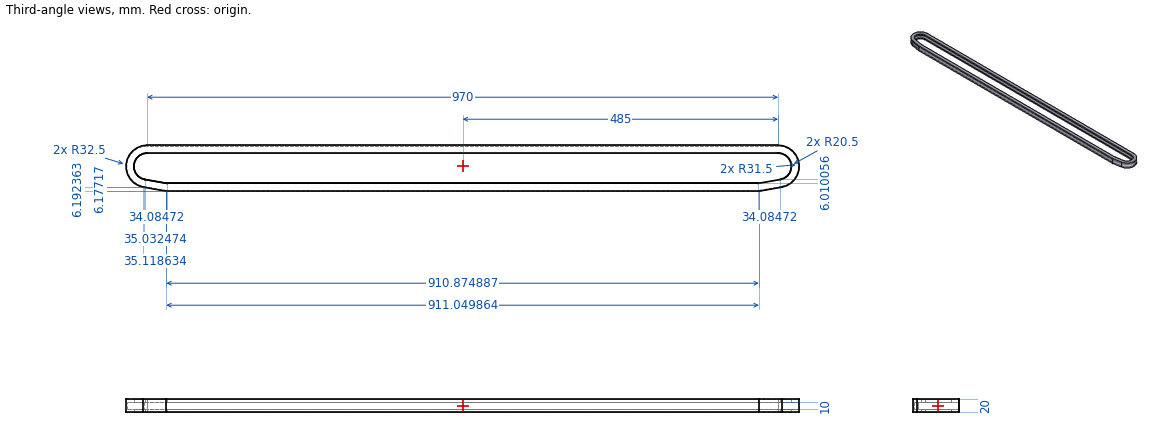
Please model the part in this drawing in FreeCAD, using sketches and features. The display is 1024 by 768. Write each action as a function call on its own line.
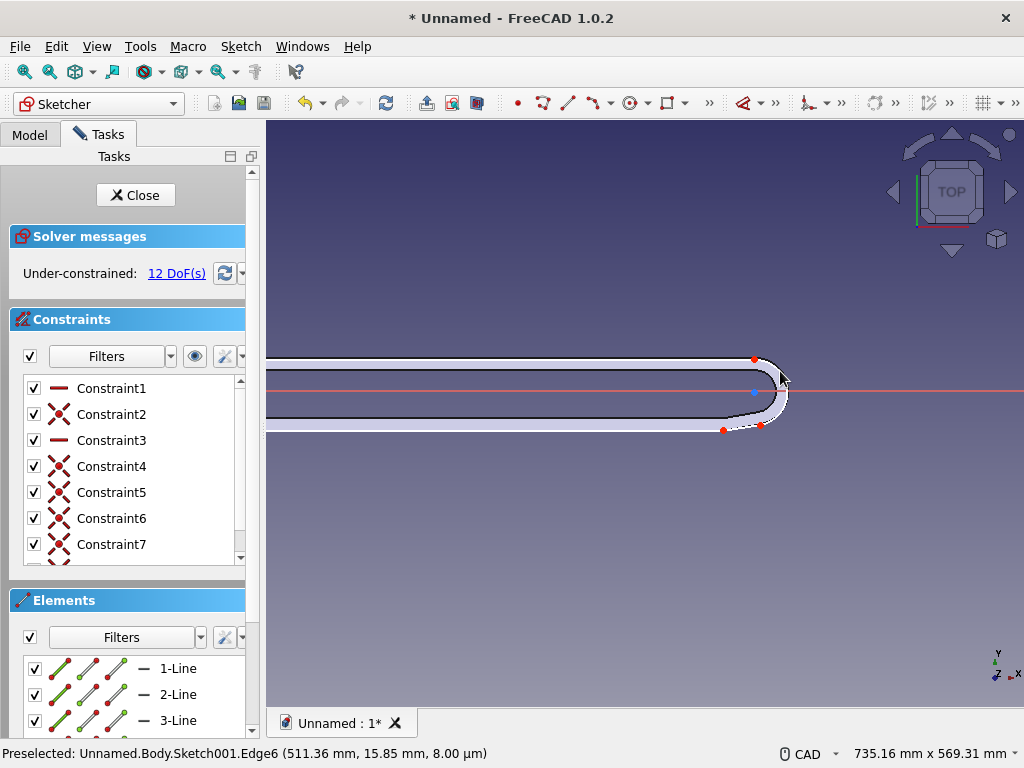
click(455, 360)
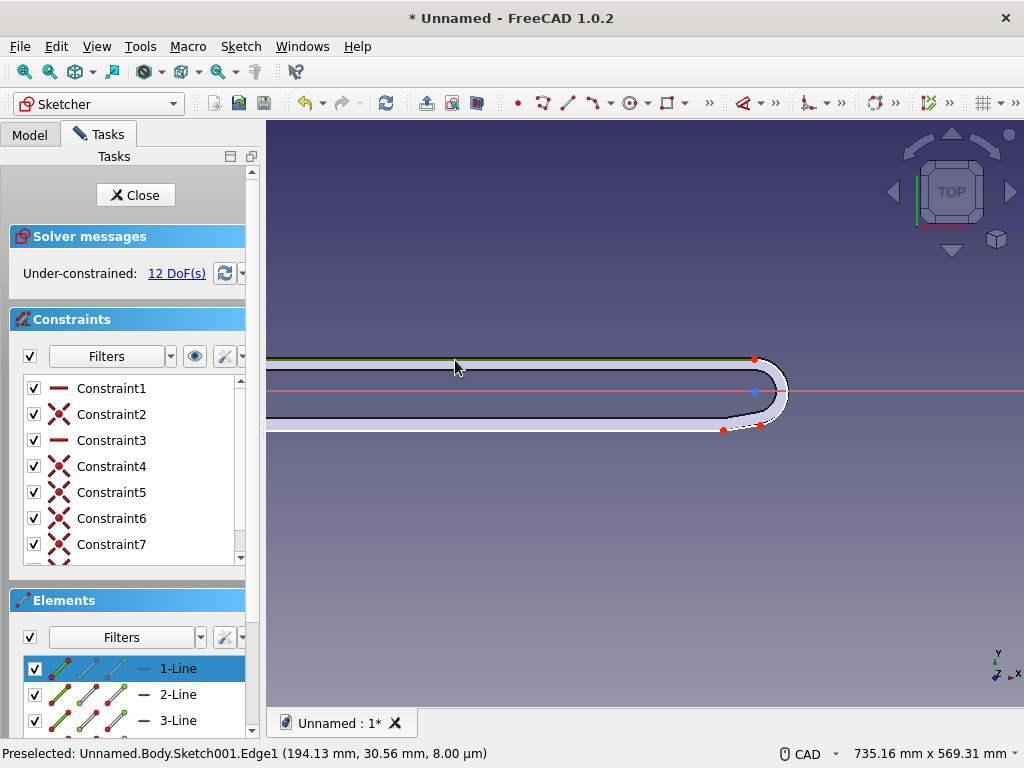
scroll(764, 425, down, 5)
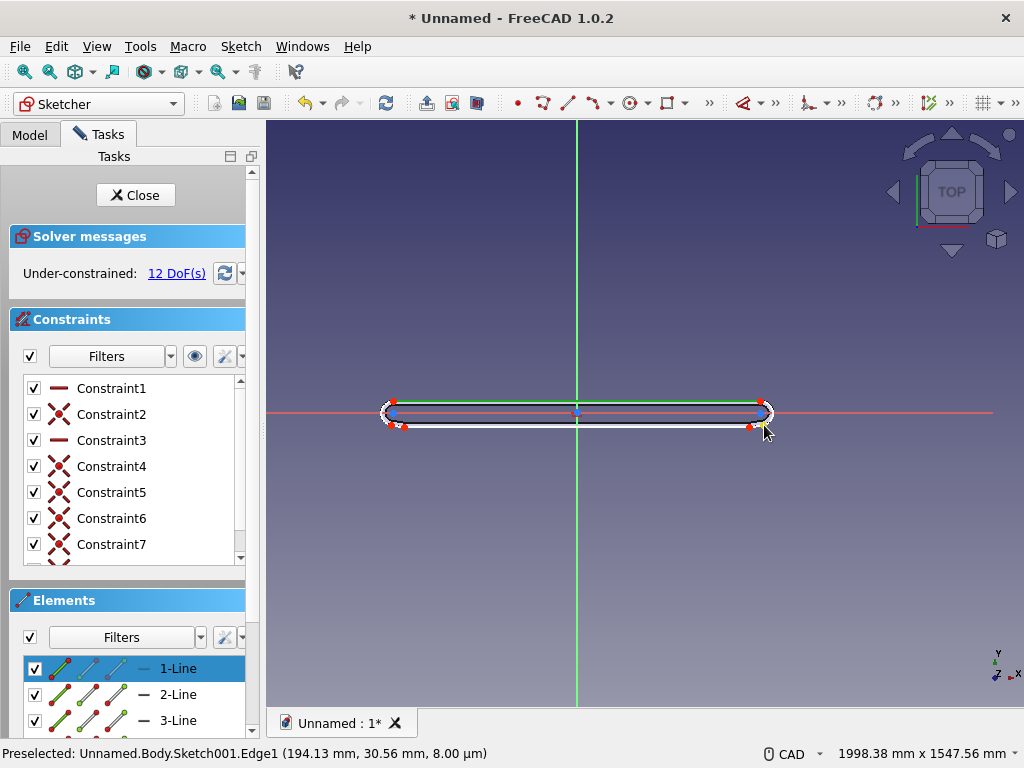
scroll(384, 406, up, 4)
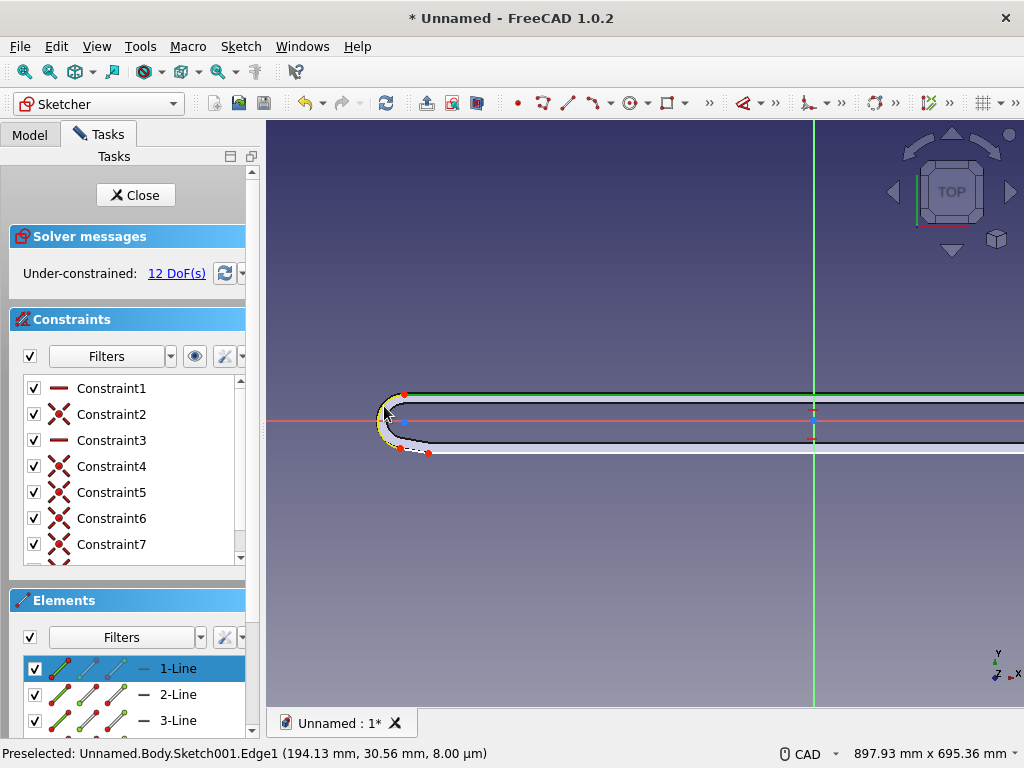
click(384, 405)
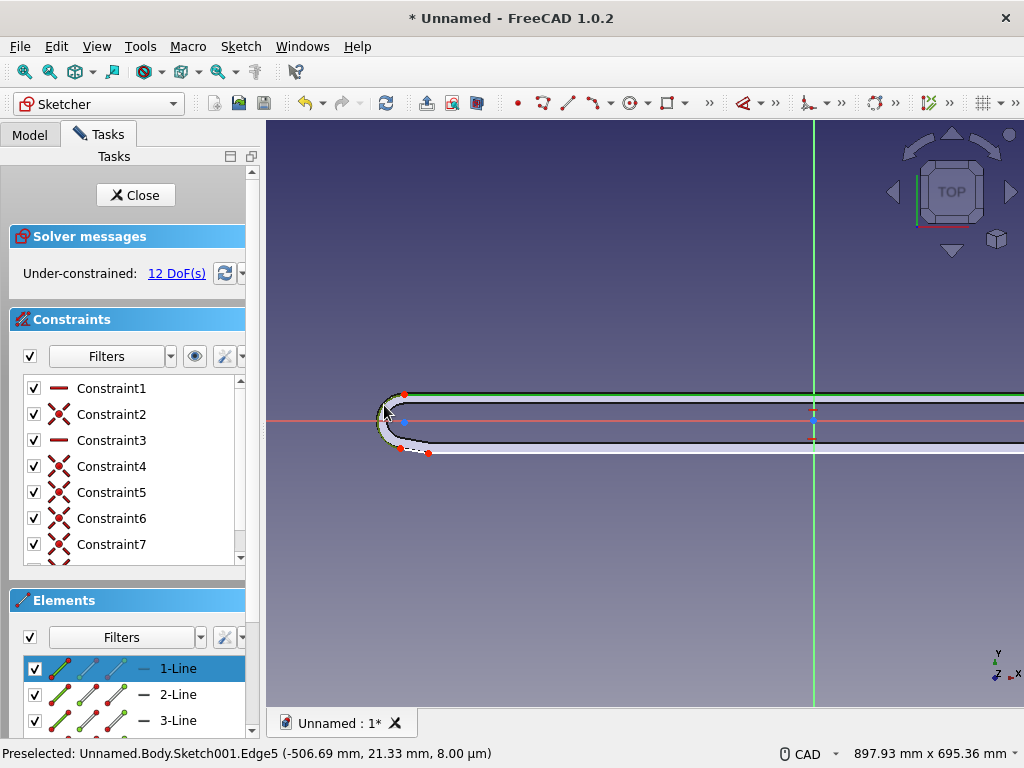
key(t)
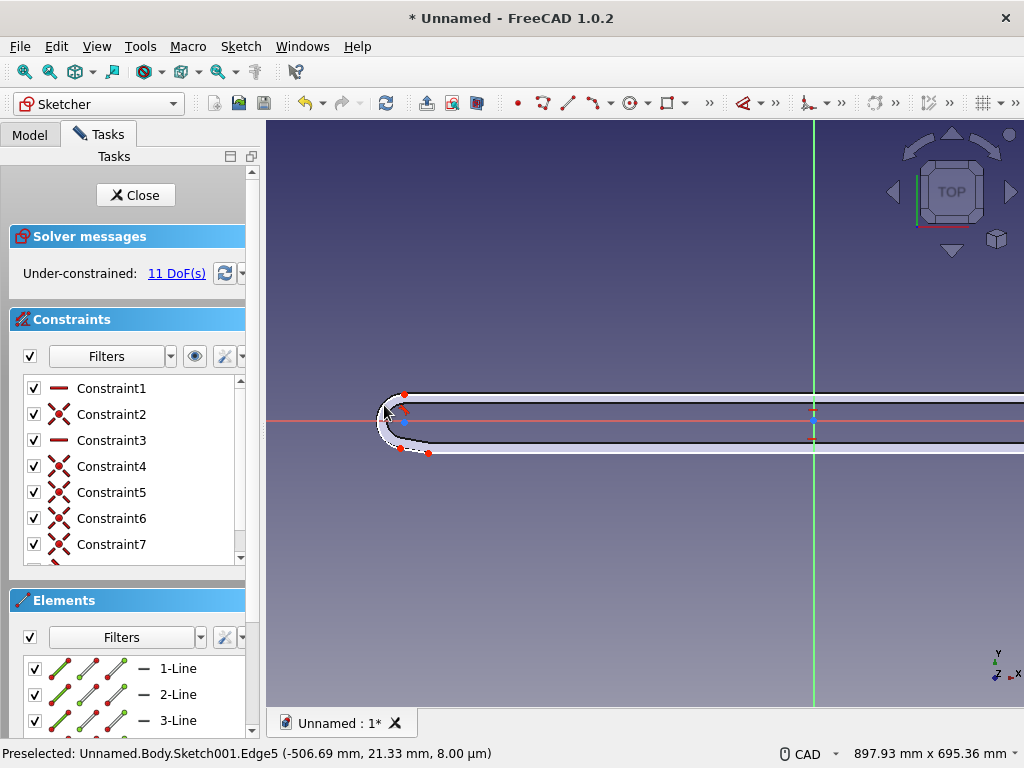
click(650, 395)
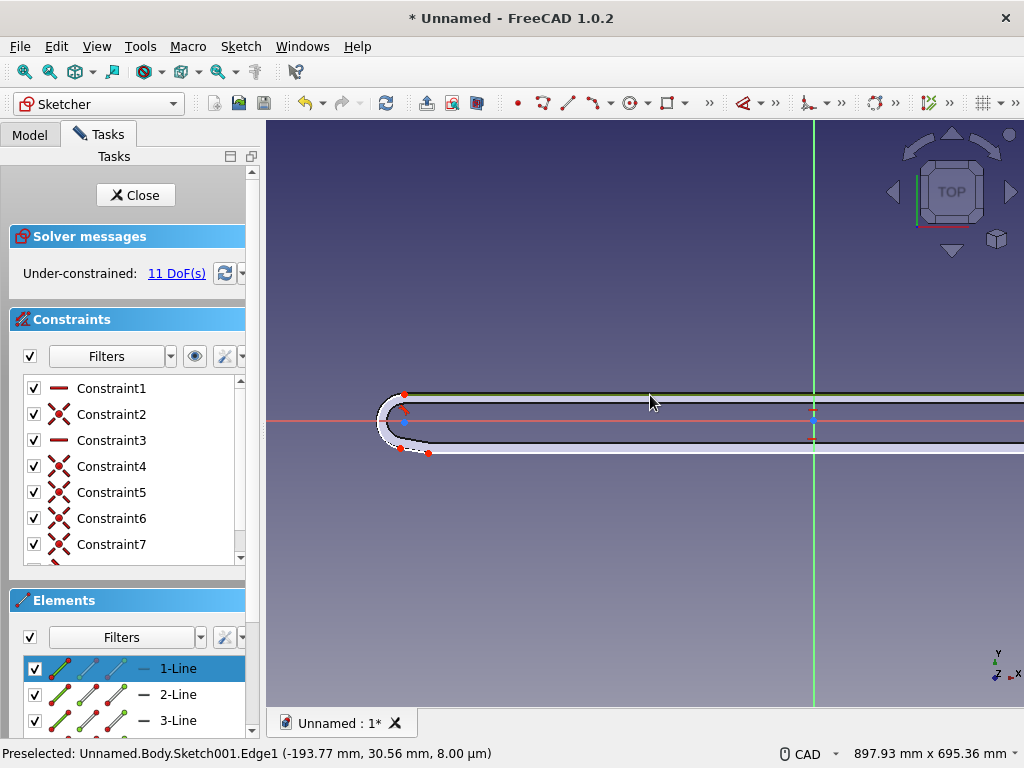
scroll(383, 406, down, 4)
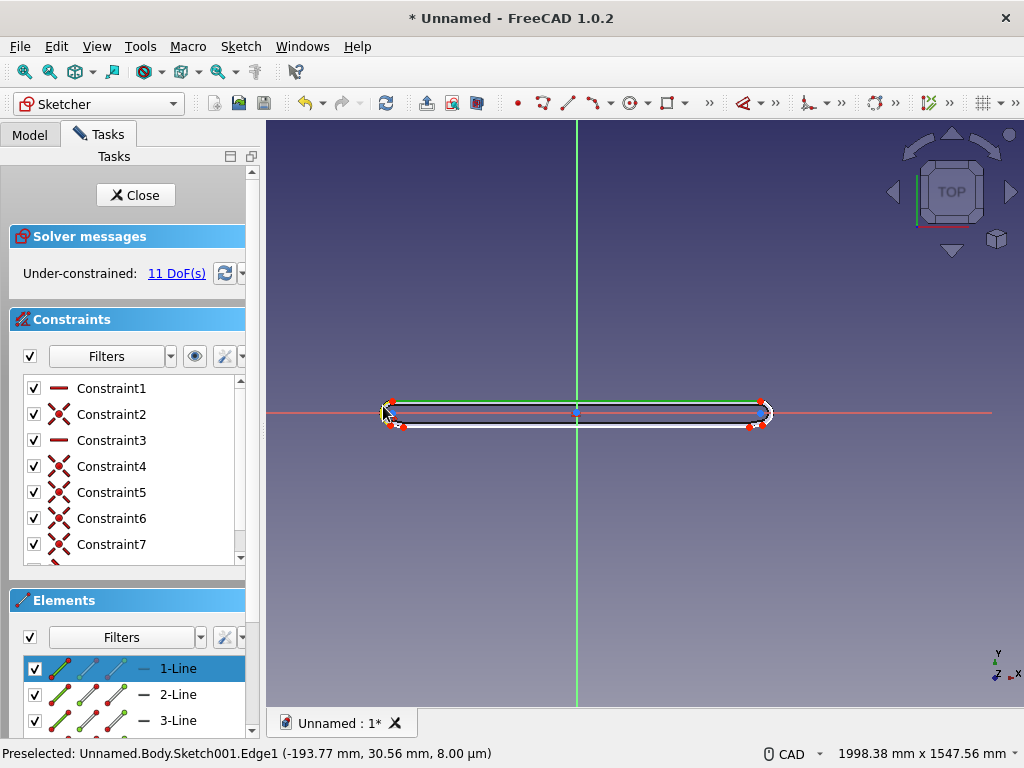
scroll(771, 419, up, 4)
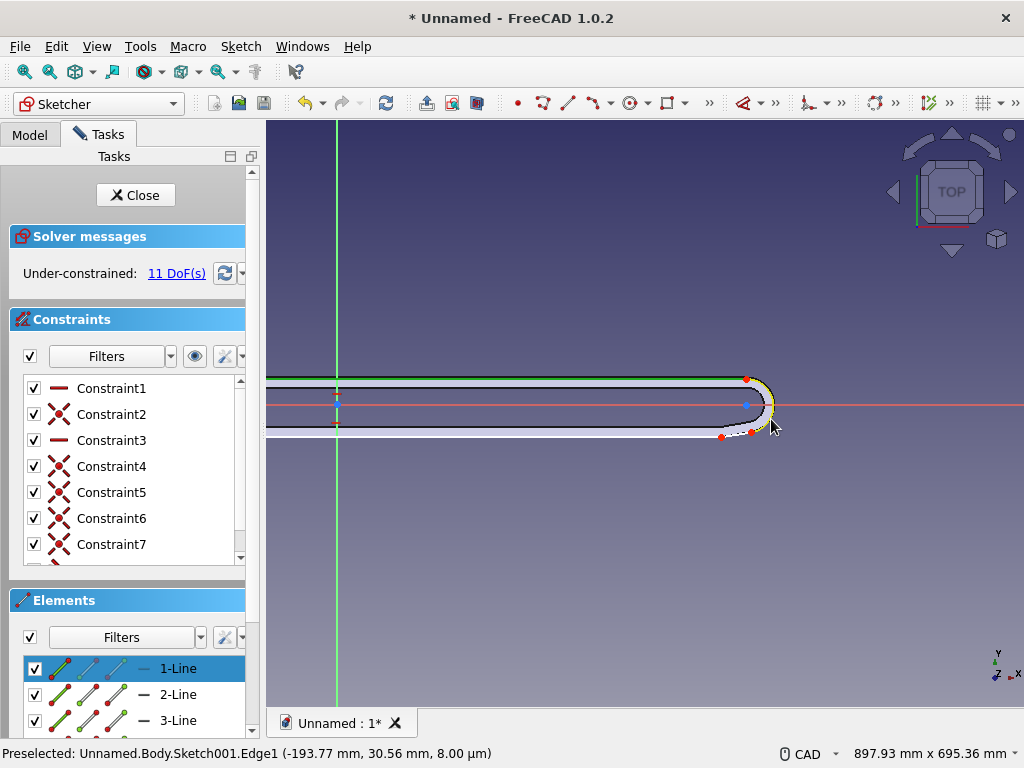
click(770, 419)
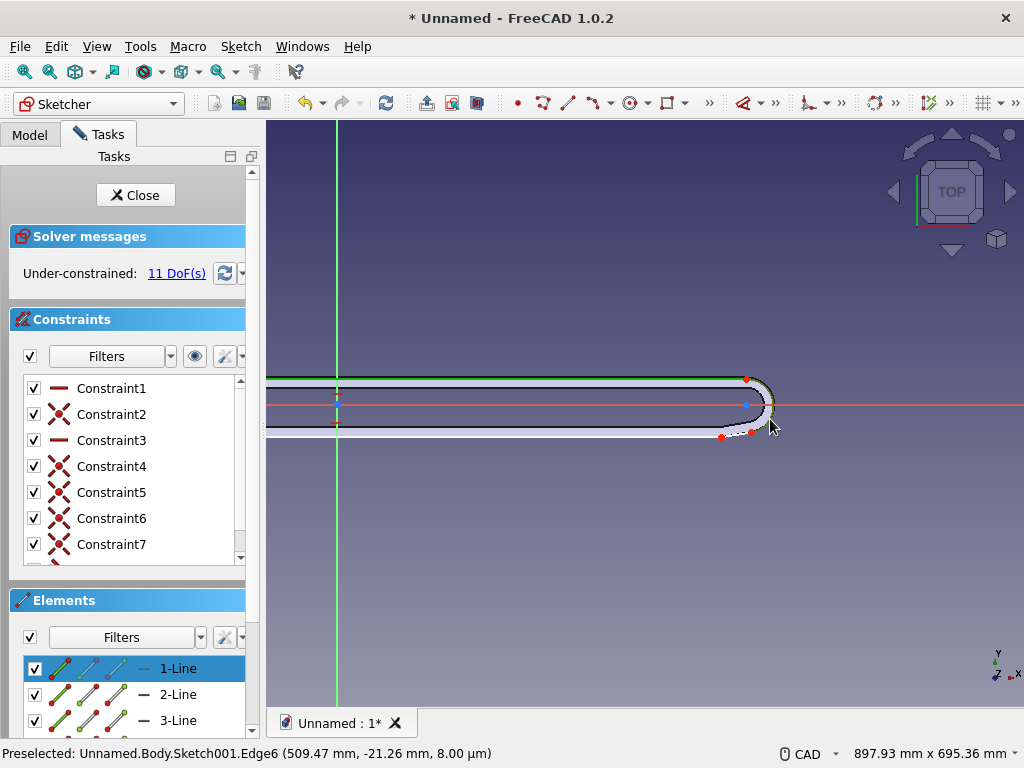
key(t)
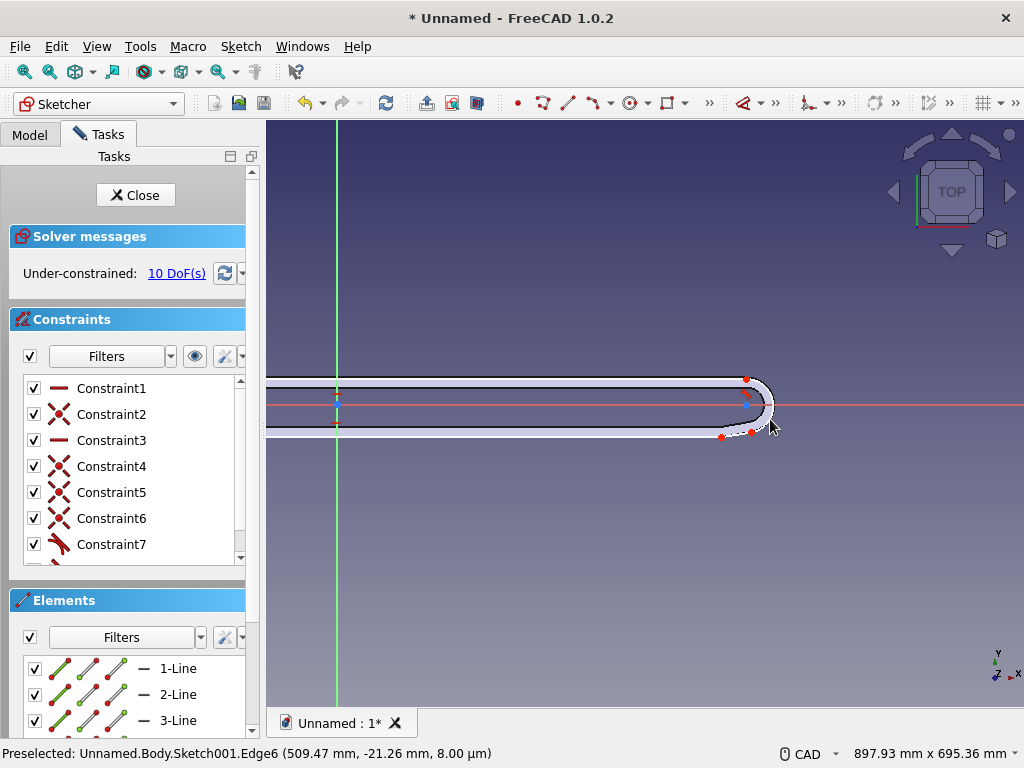
scroll(772, 419, down, 4)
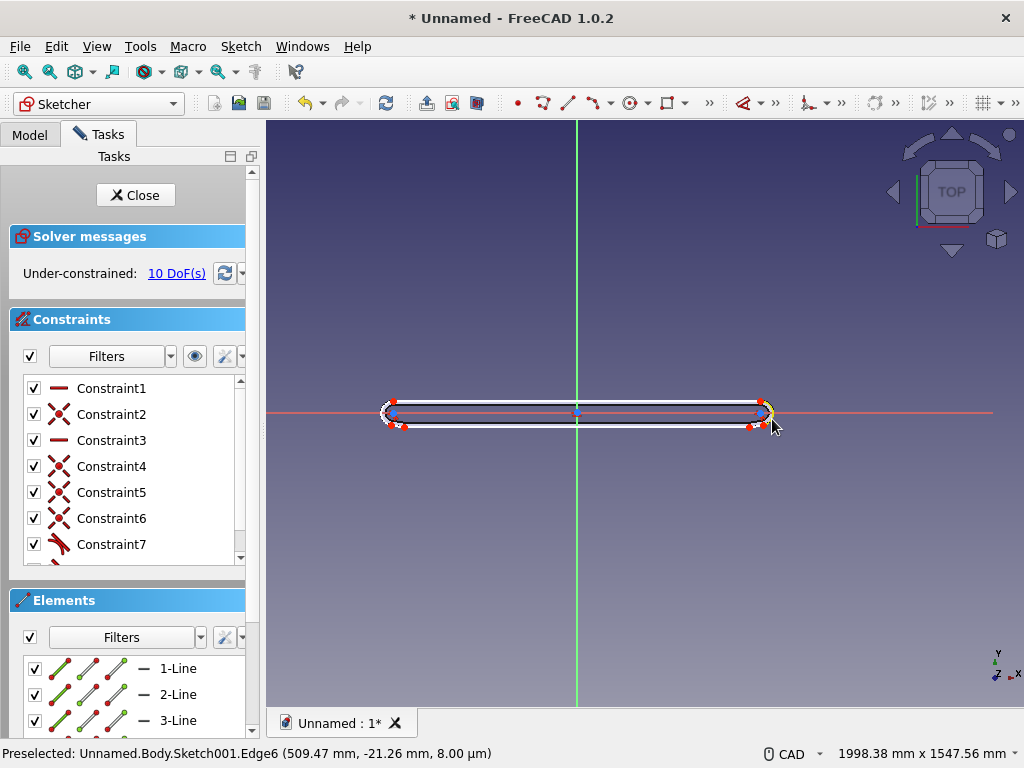
scroll(396, 426, up, 5)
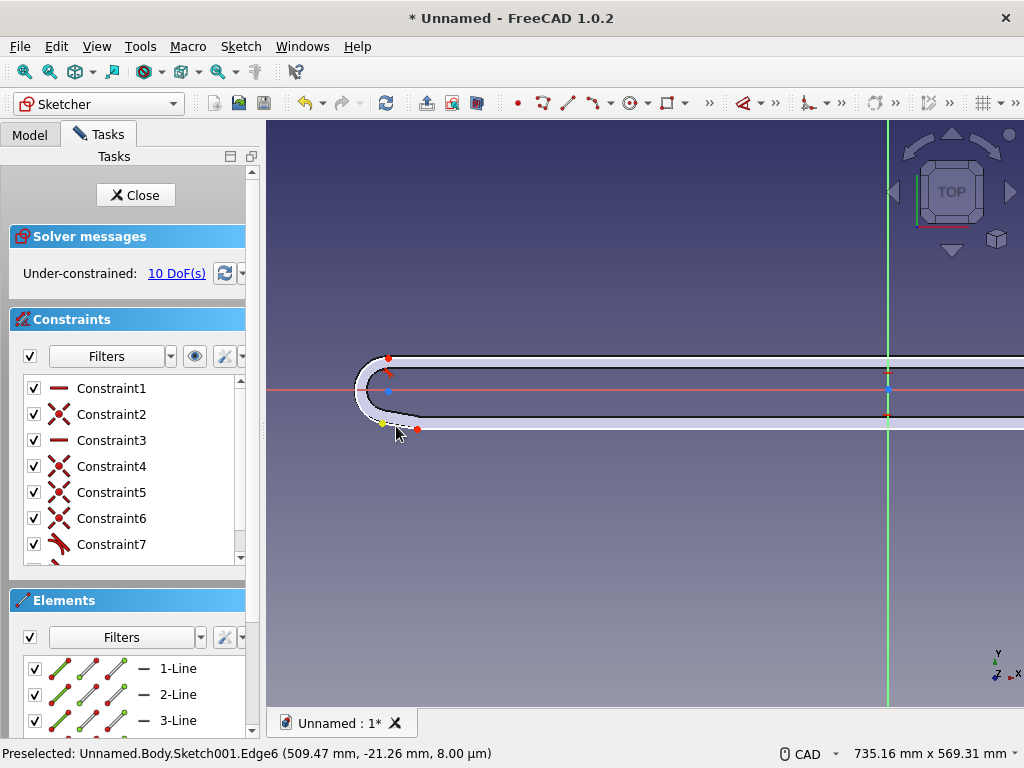
click(397, 426)